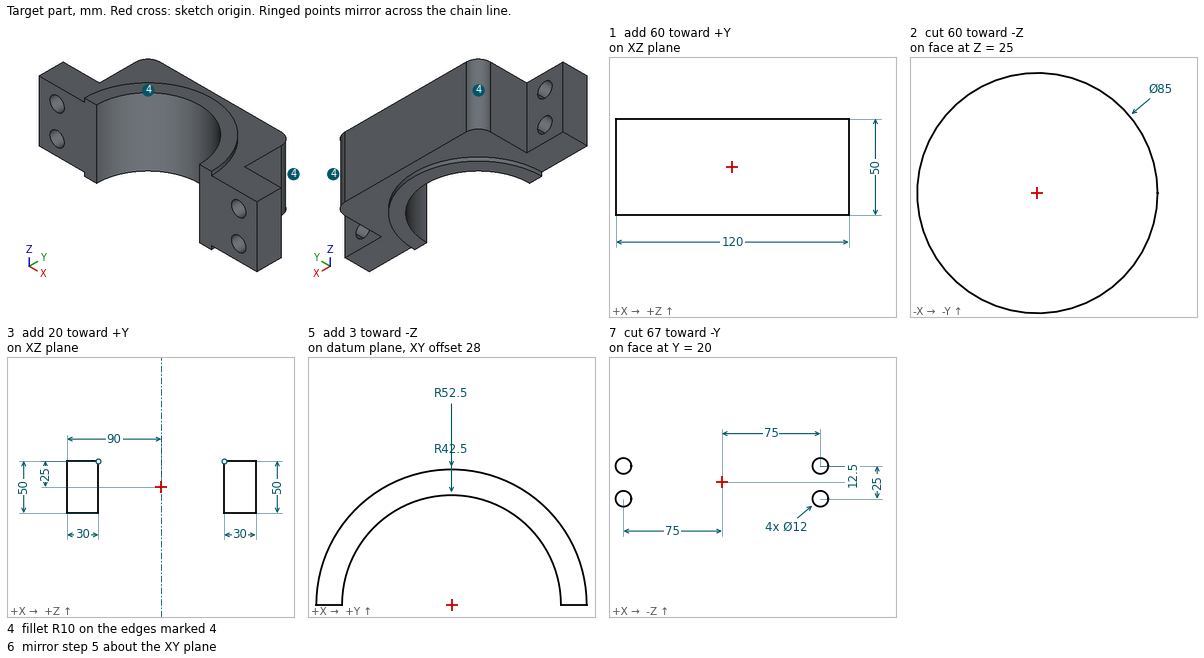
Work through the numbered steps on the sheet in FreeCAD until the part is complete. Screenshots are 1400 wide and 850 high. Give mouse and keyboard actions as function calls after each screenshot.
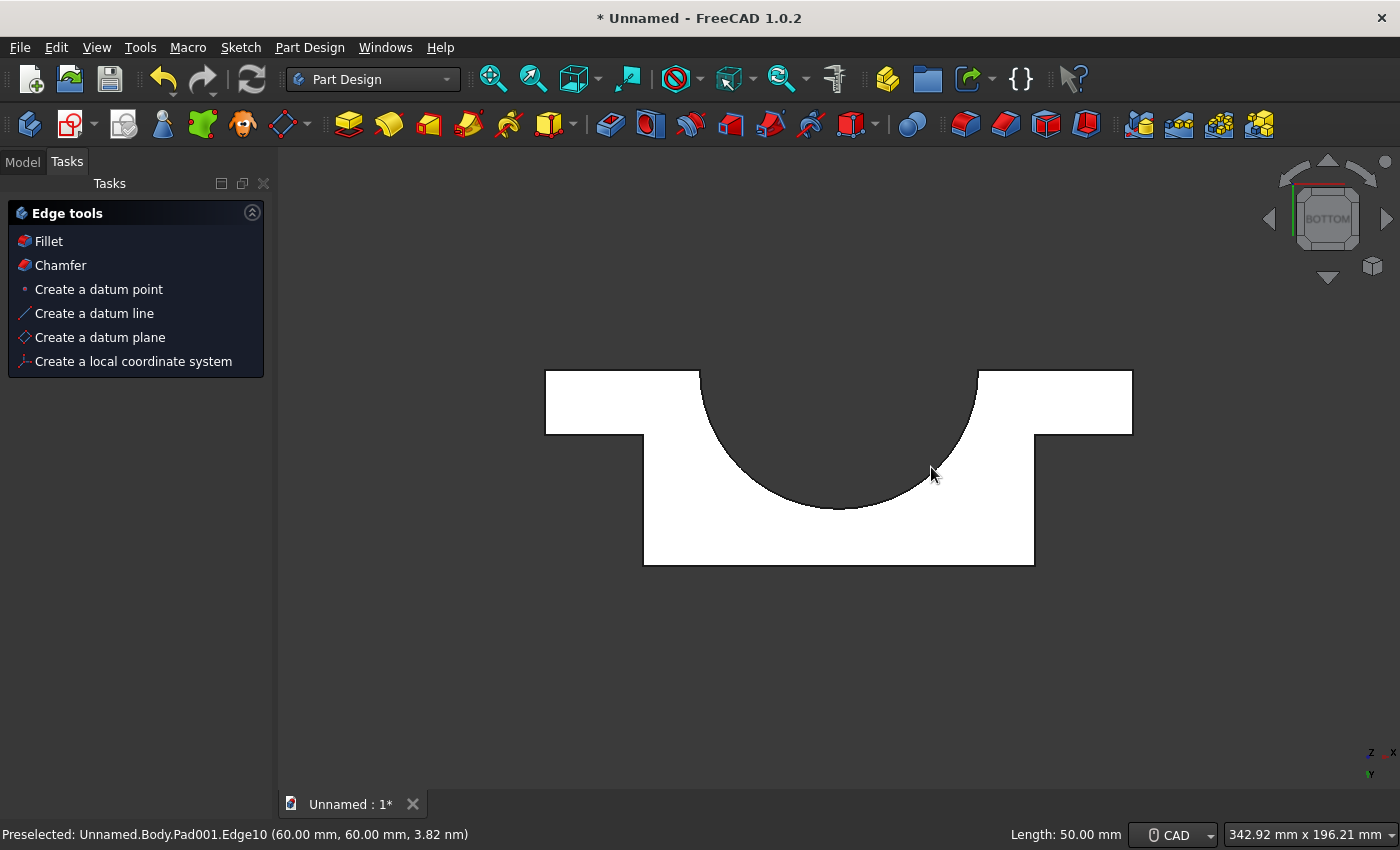
key(4)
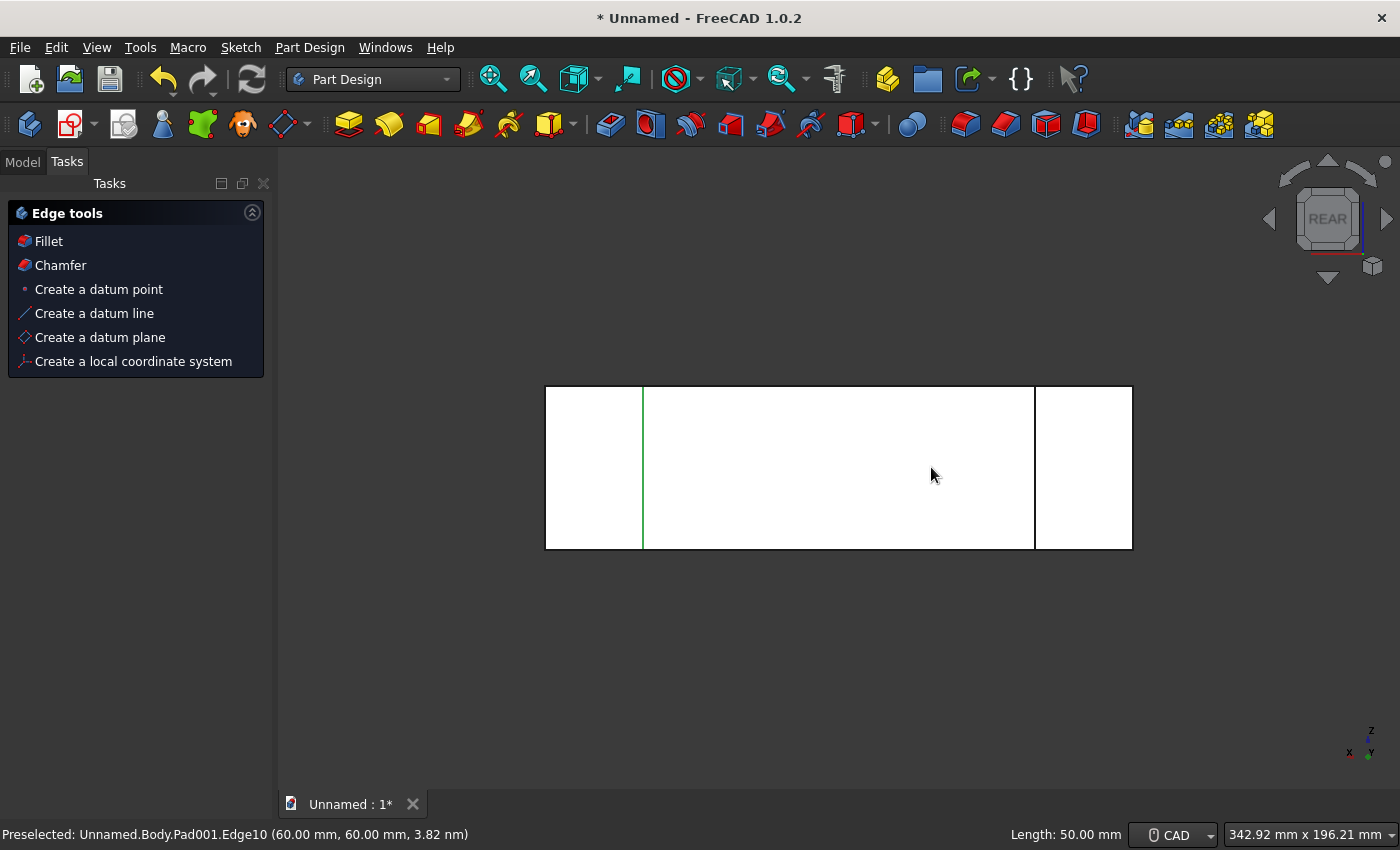
click(1035, 467, ctrl)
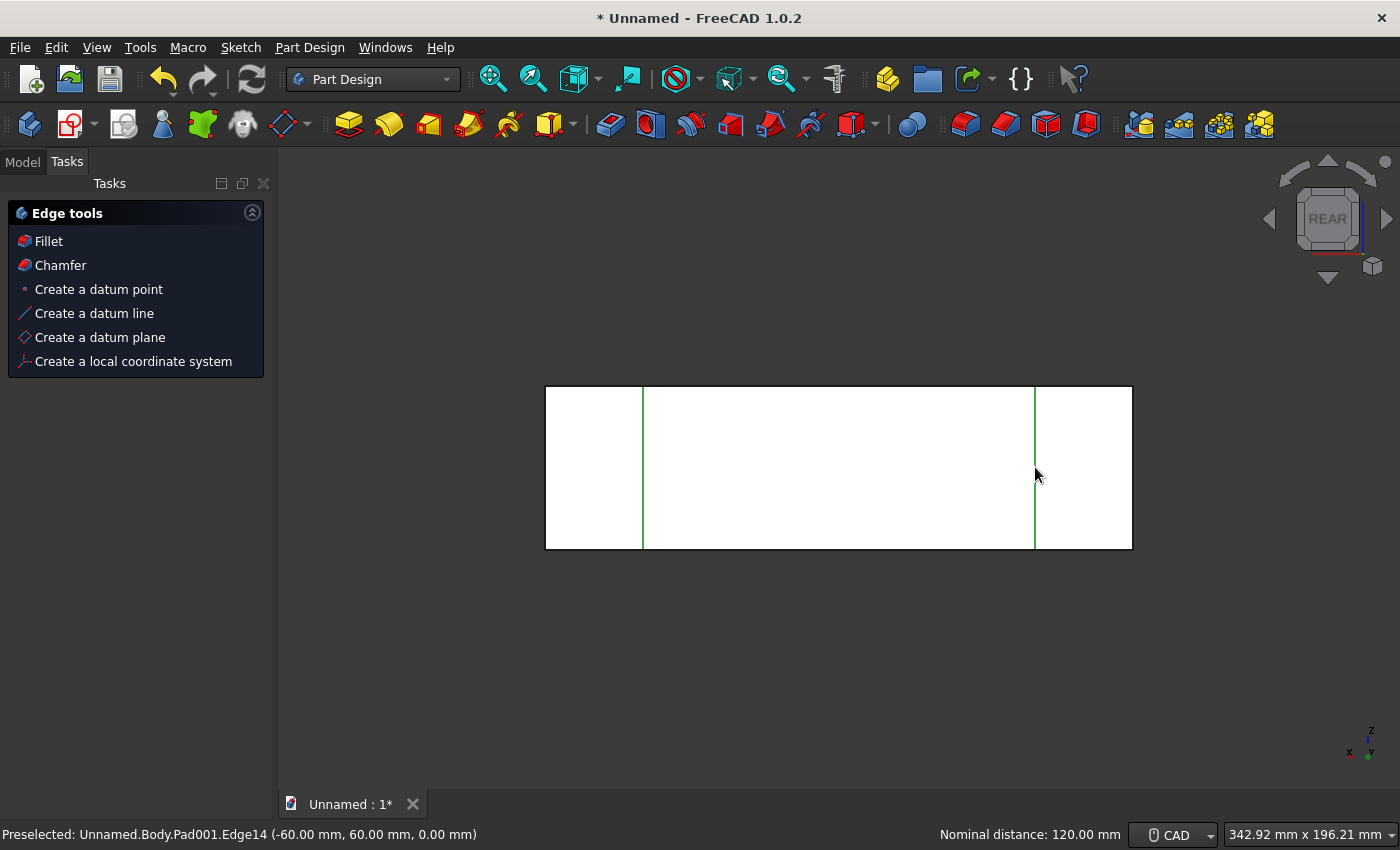
click(966, 124)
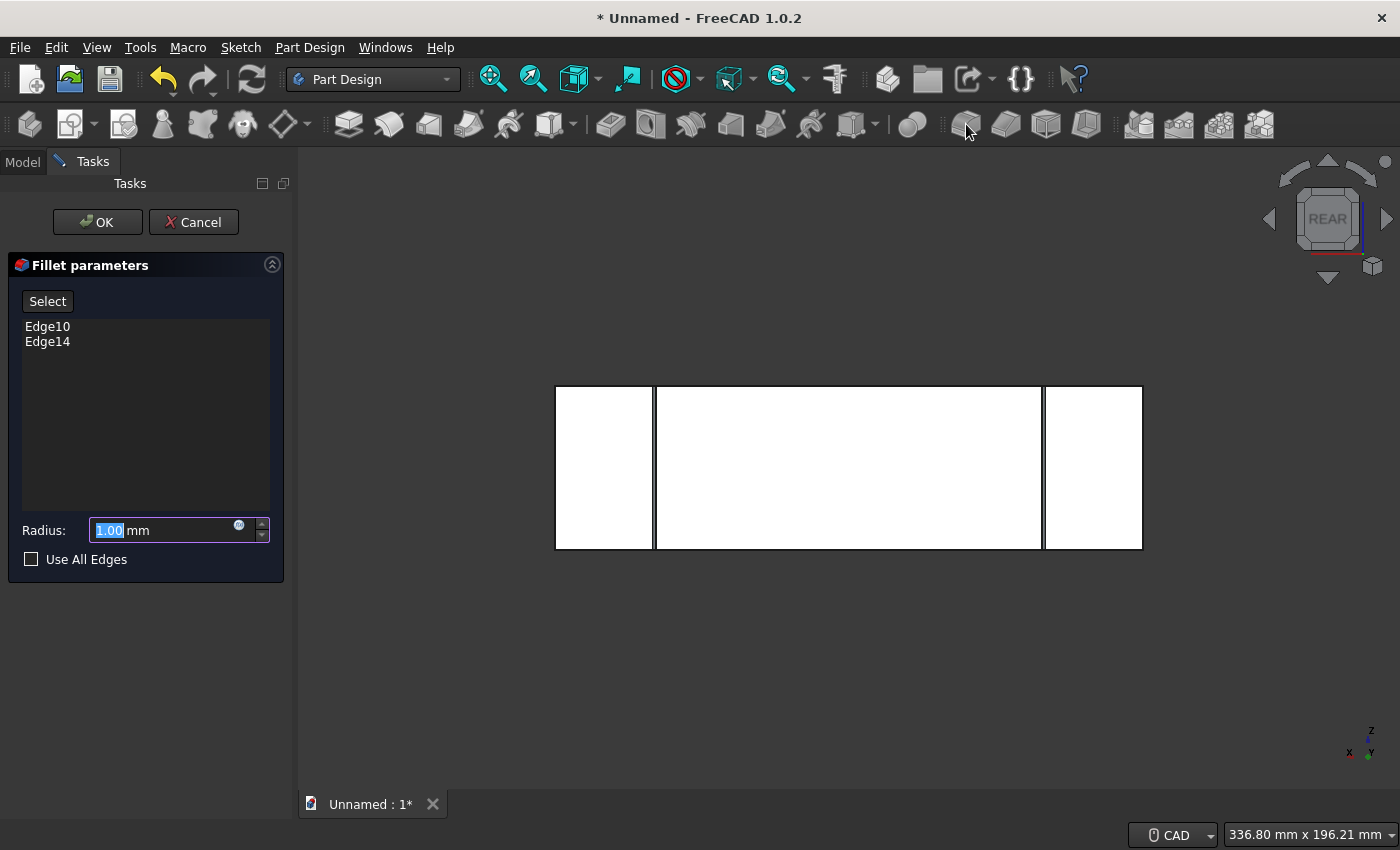
text(10)
key(Tab)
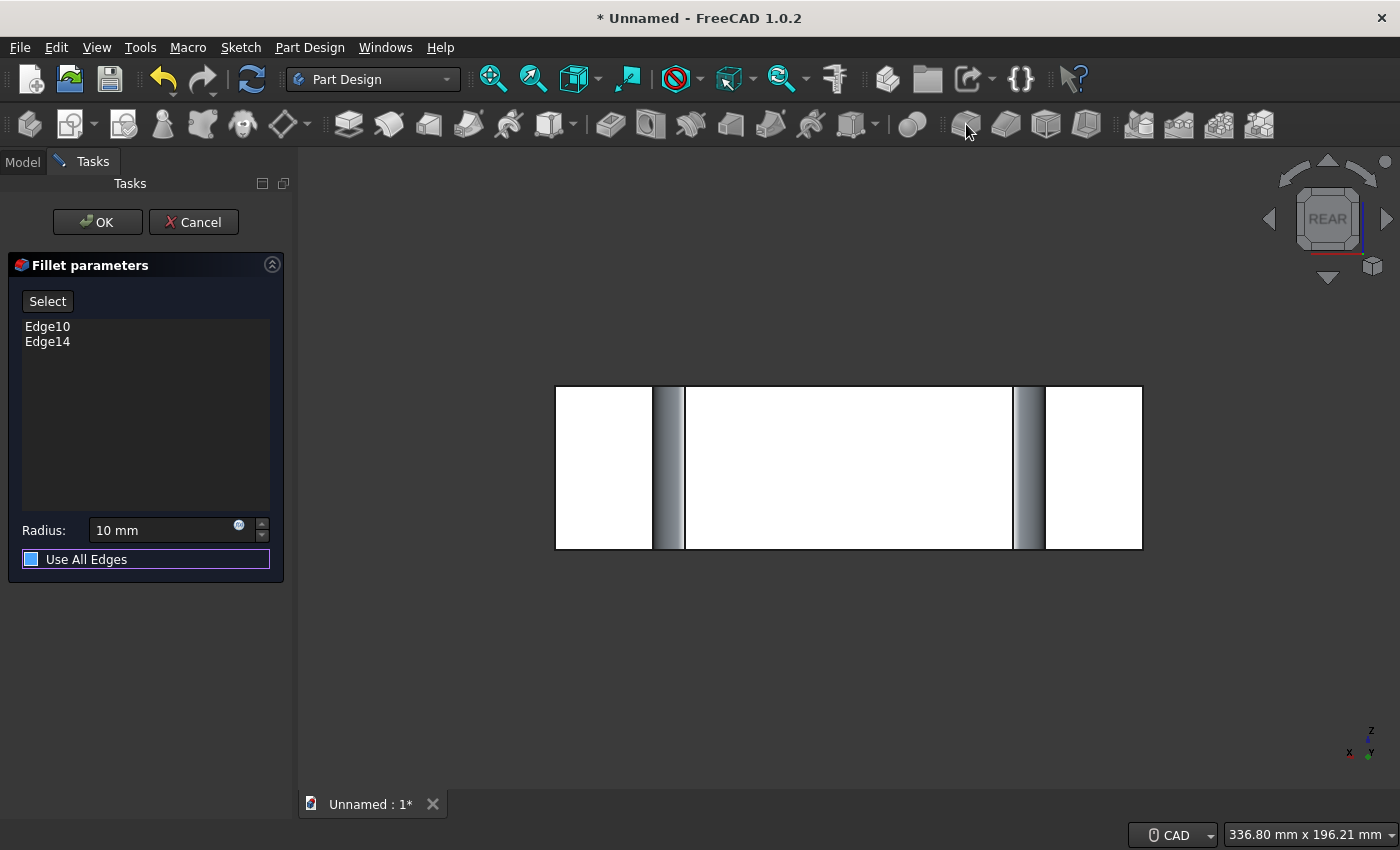
click(98, 222)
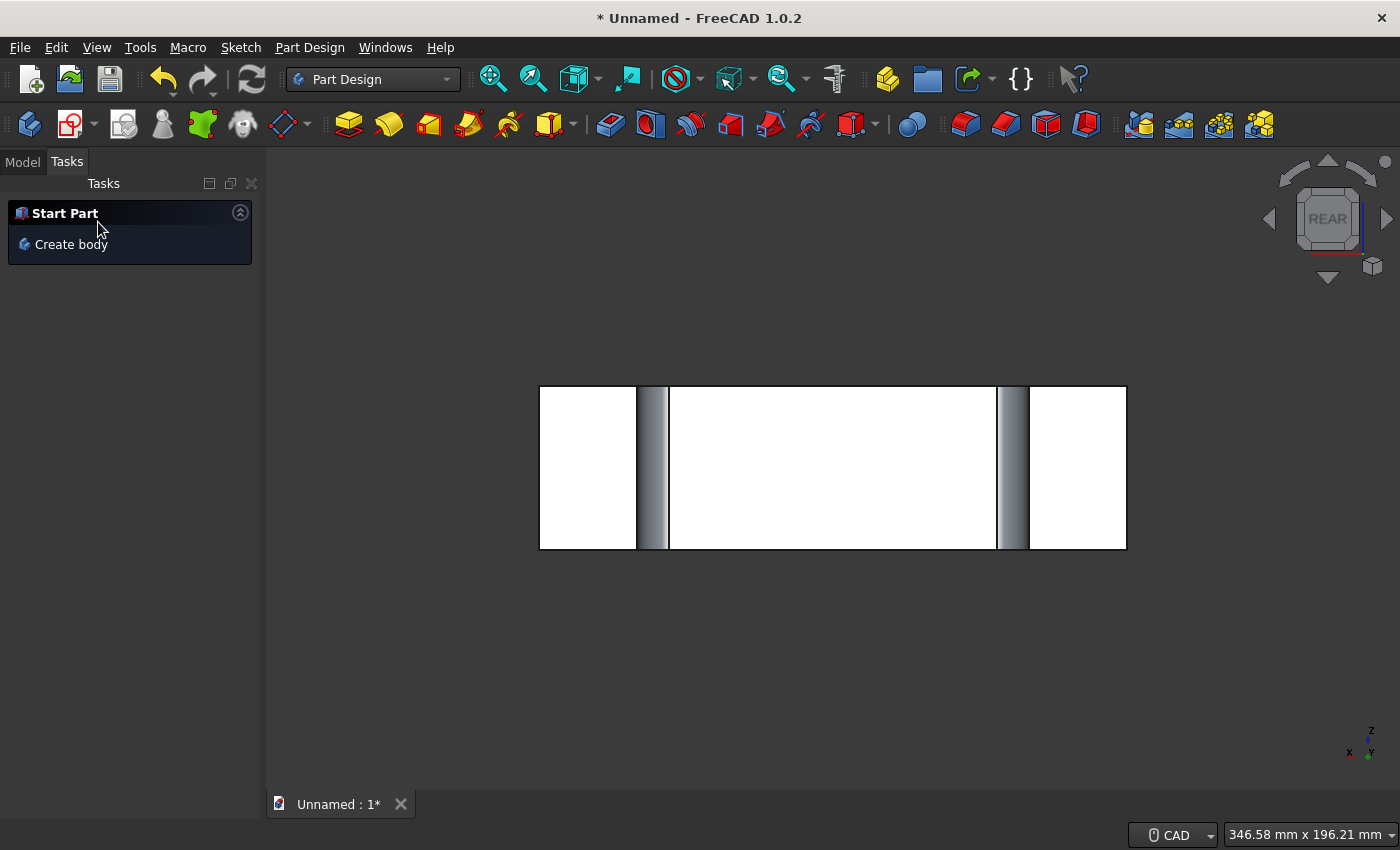
click(23, 161)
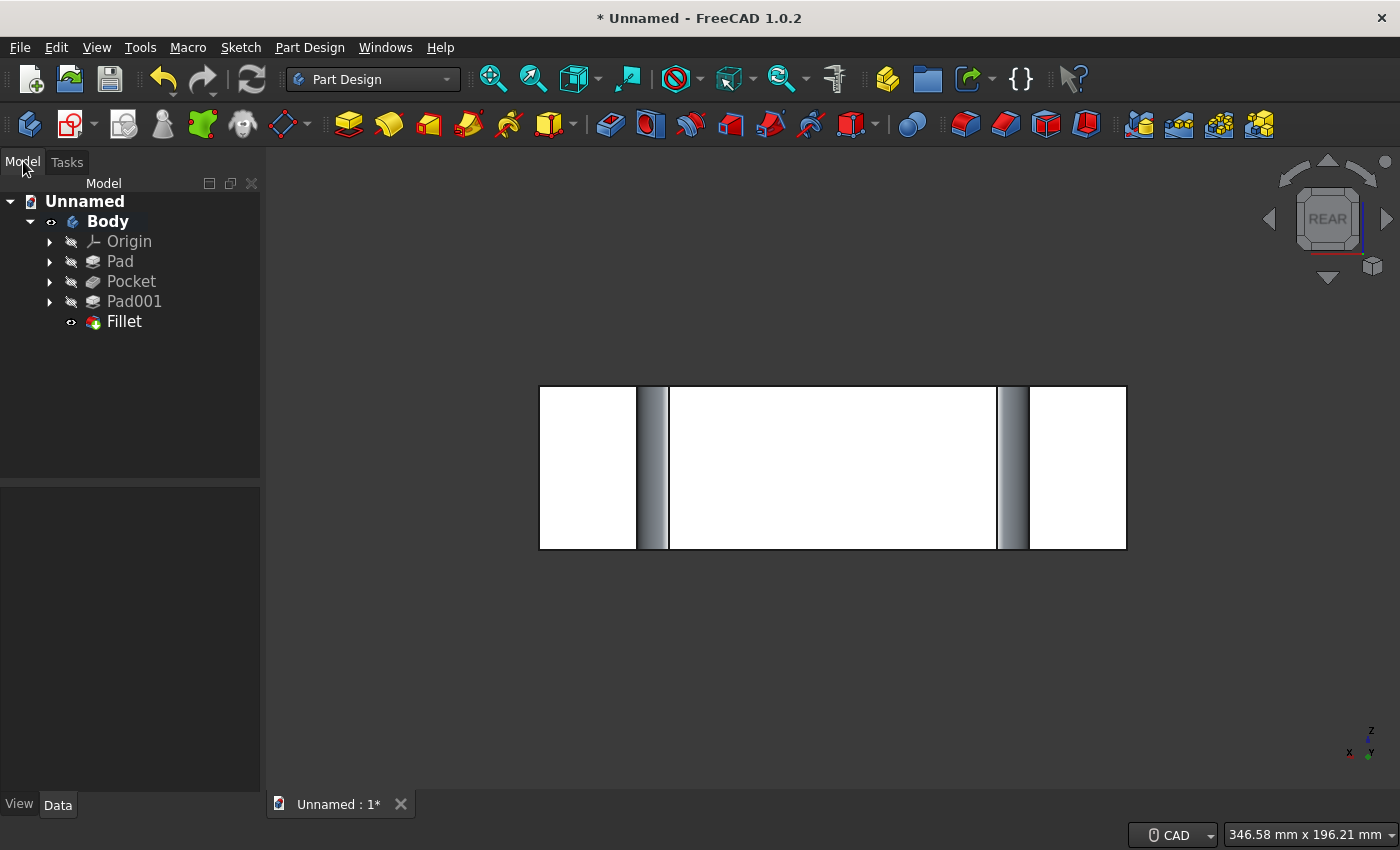
click(50, 242)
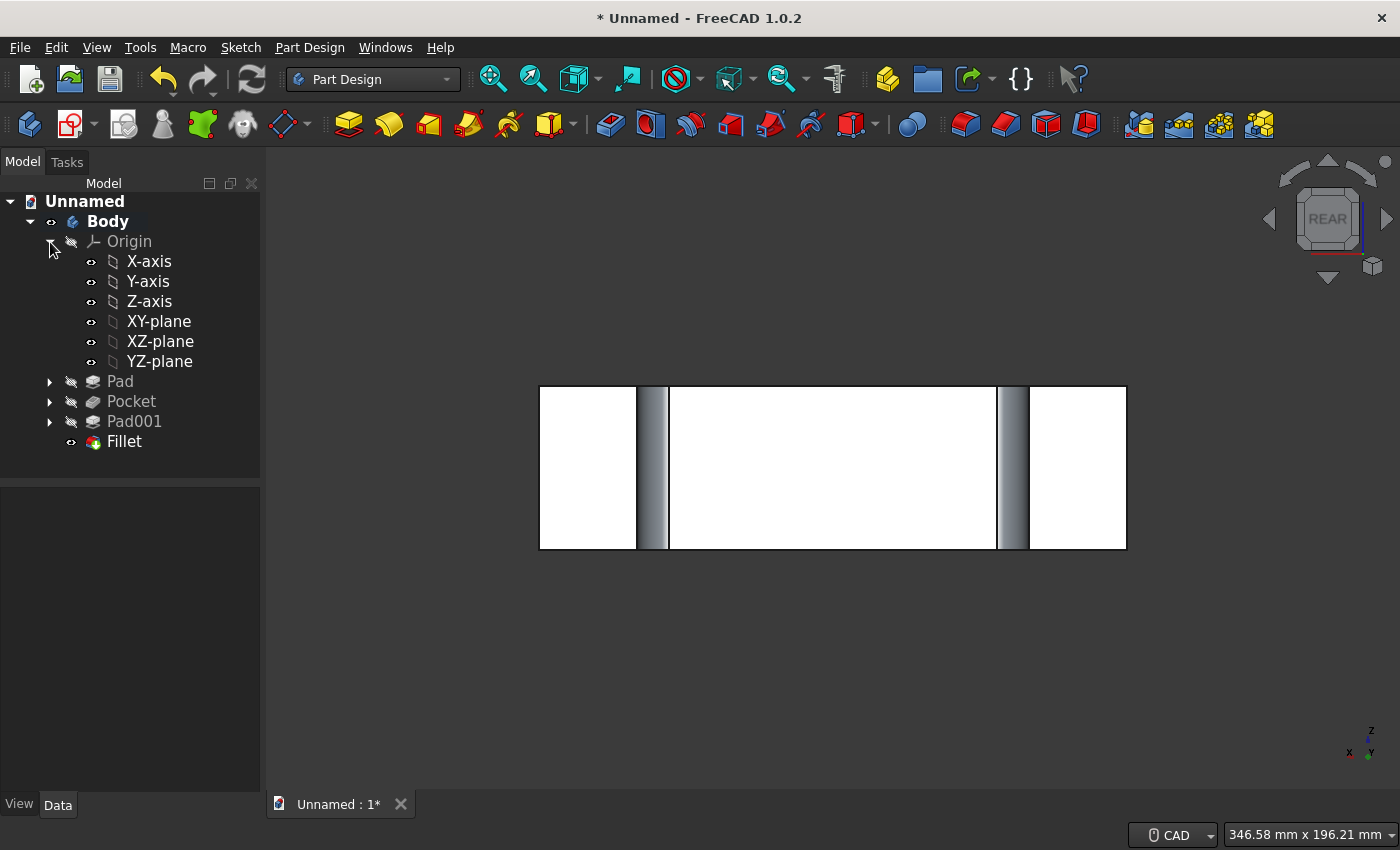
click(136, 322)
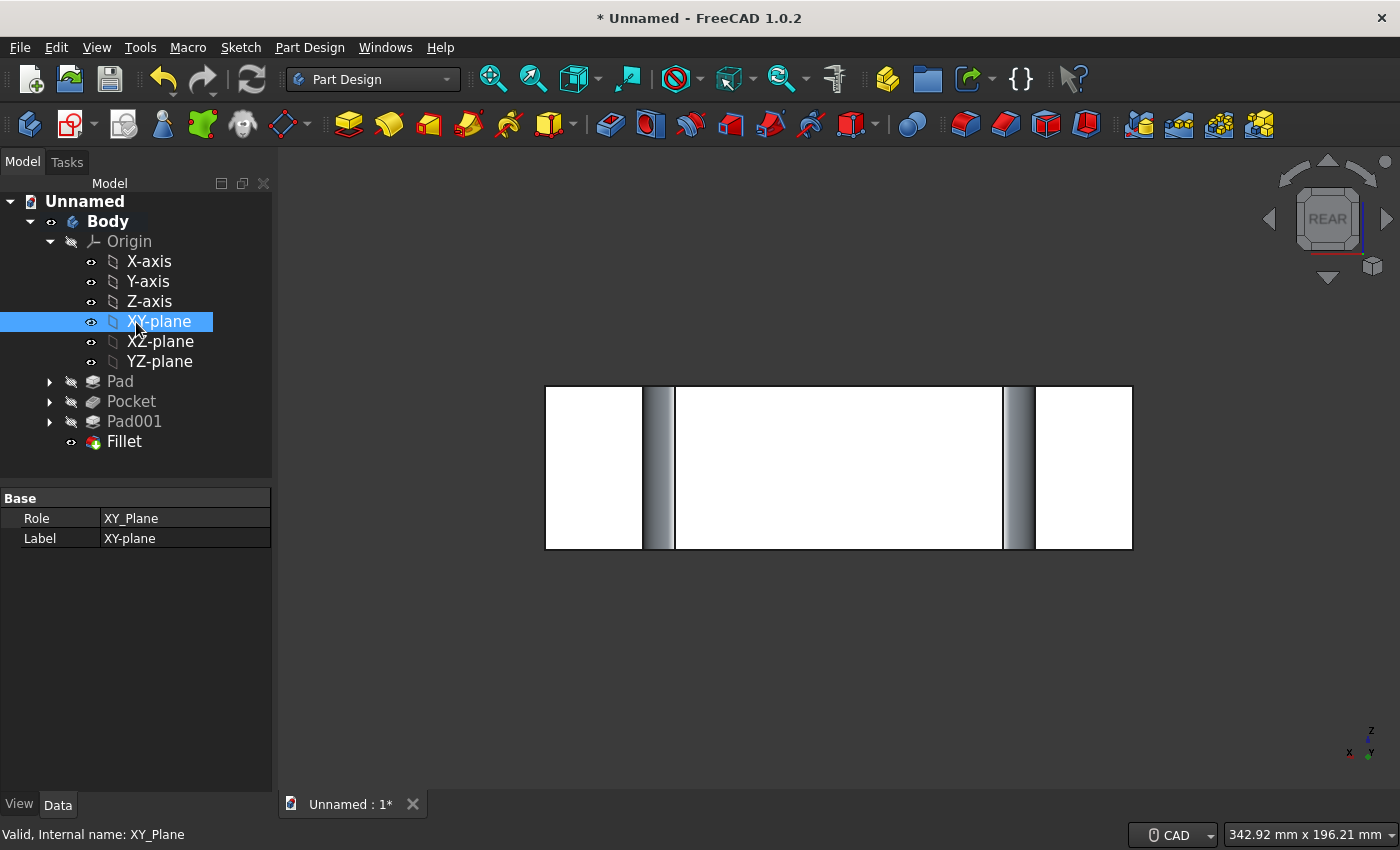
click(284, 124)